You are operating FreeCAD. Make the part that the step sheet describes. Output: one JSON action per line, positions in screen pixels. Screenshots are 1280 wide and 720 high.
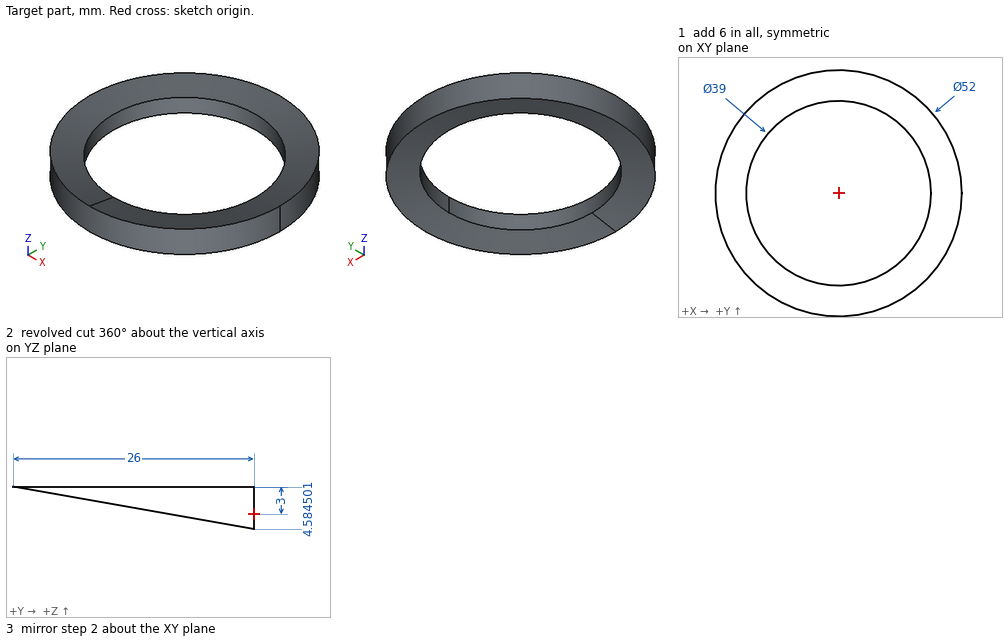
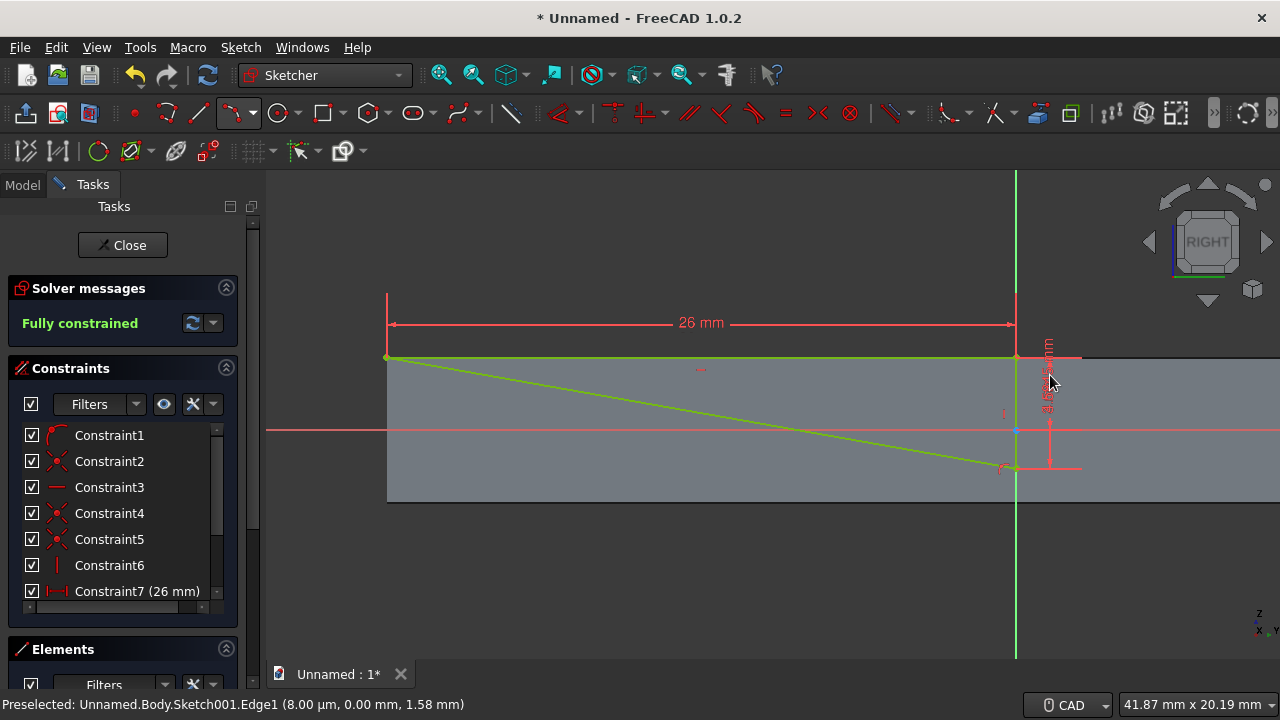
{"action": "left_click", "coordinate": [123, 245]}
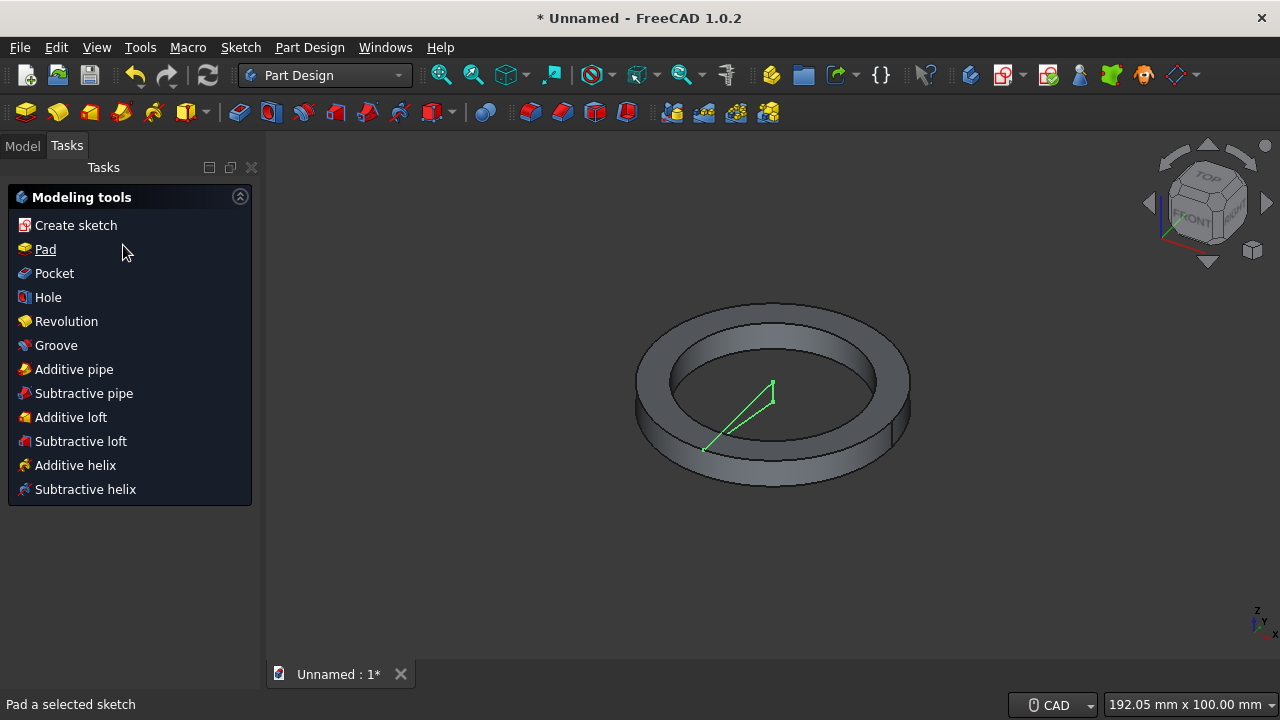
{"action": "left_click", "coordinate": [304, 112]}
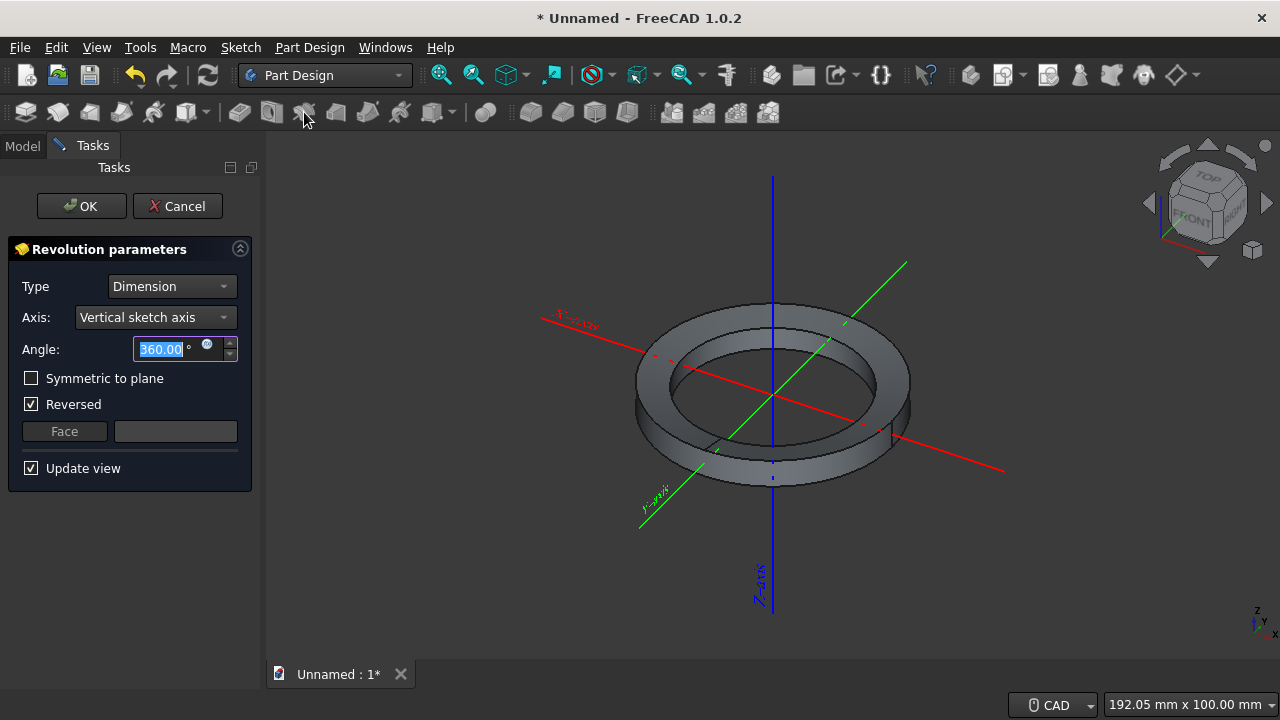
{"action": "left_click", "coordinate": [82, 206]}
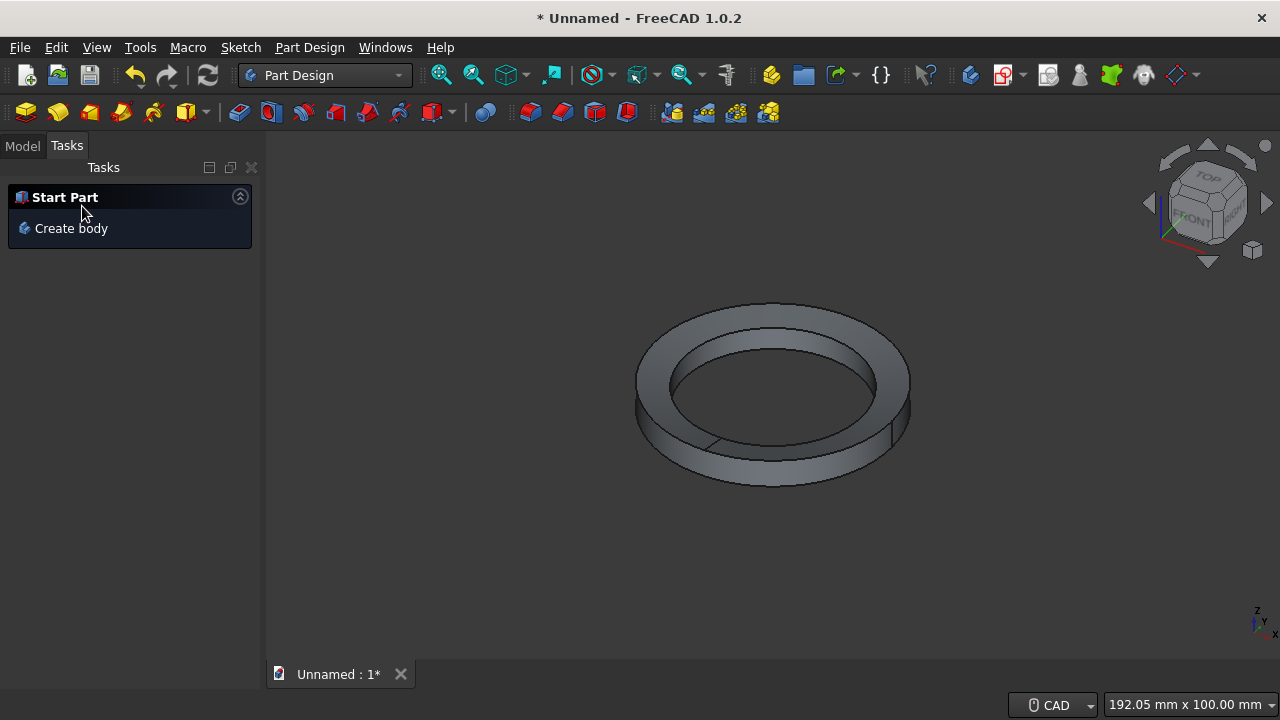
{"action": "left_click", "coordinate": [23, 145]}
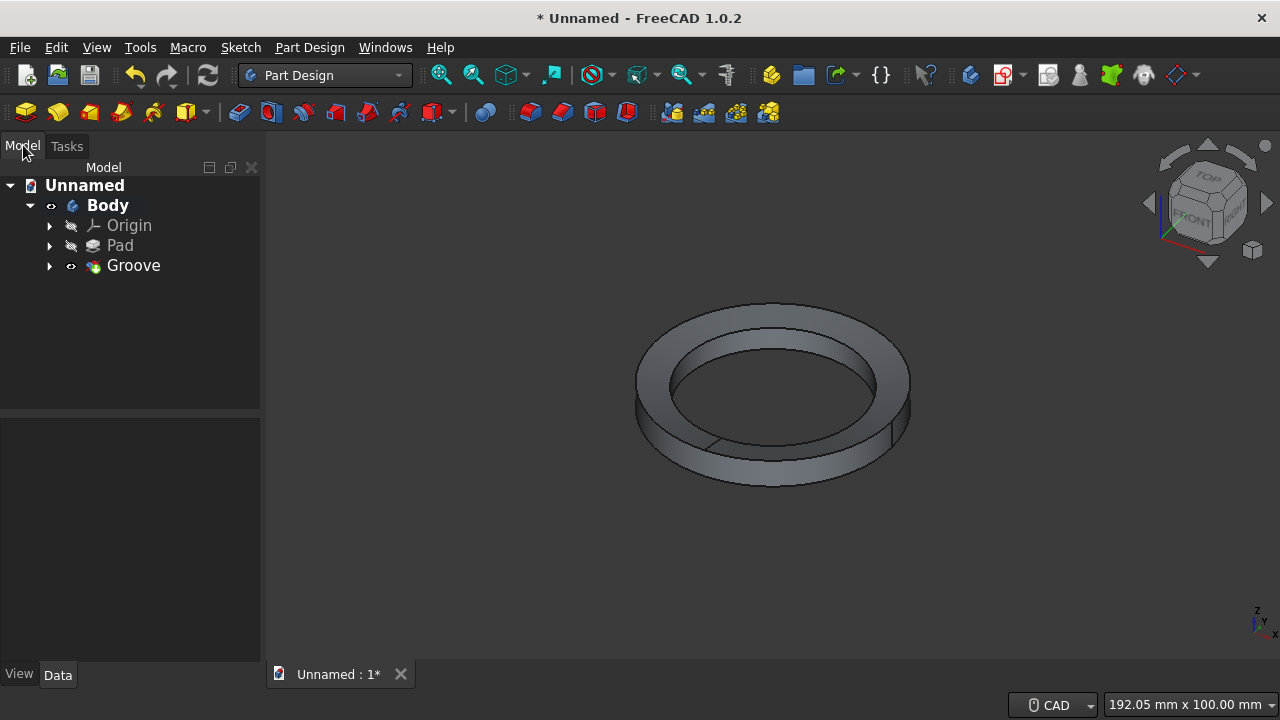
{"action": "left_click", "coordinate": [116, 266]}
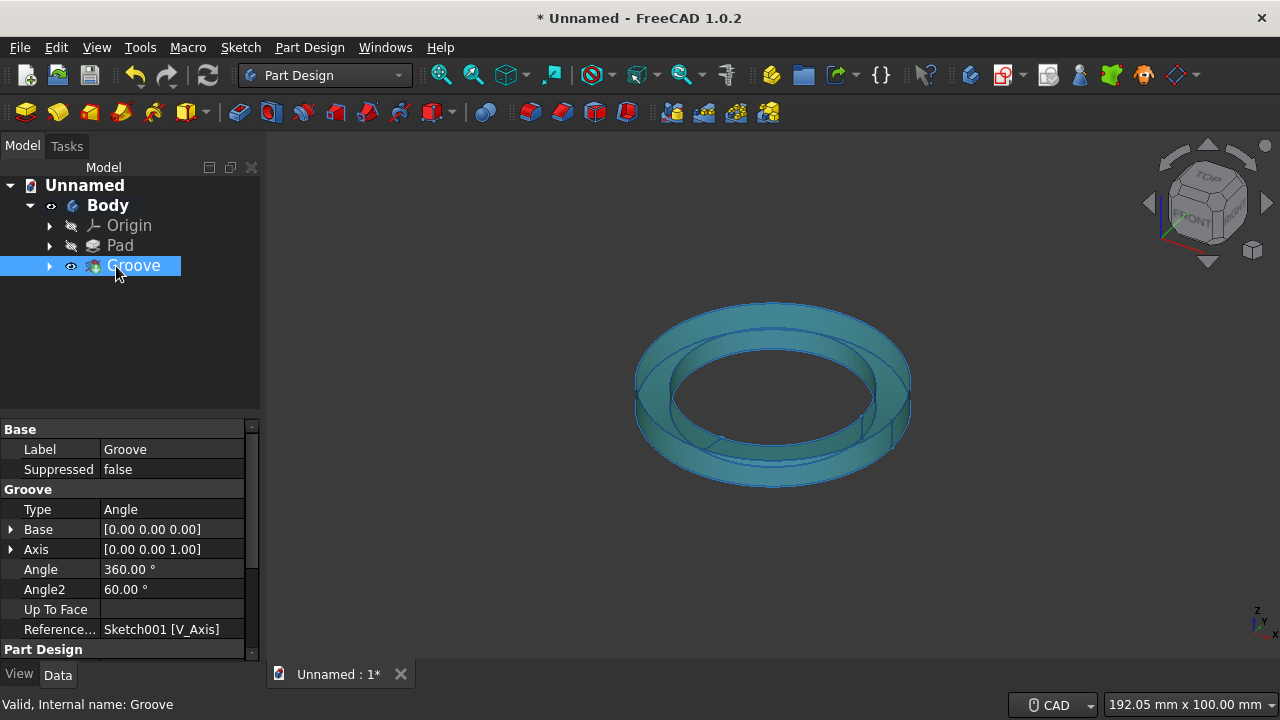
{"action": "left_click", "coordinate": [672, 112]}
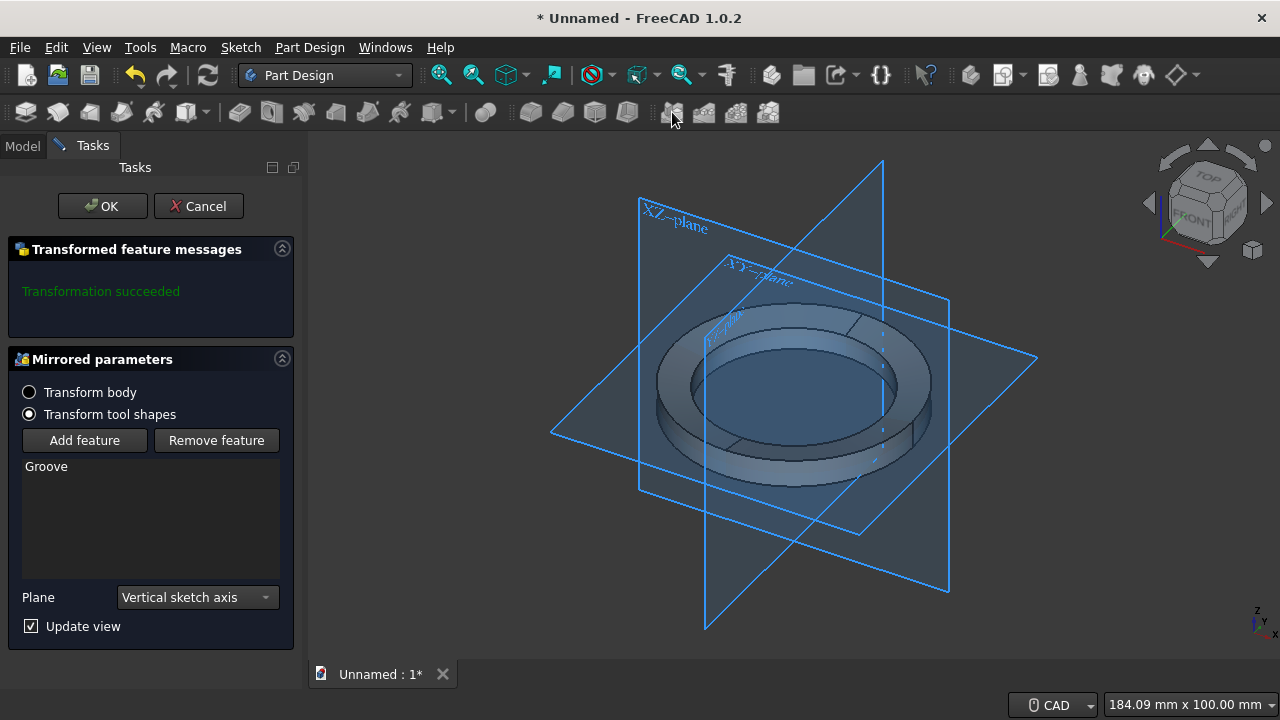
{"action": "left_click", "coordinate": [198, 598]}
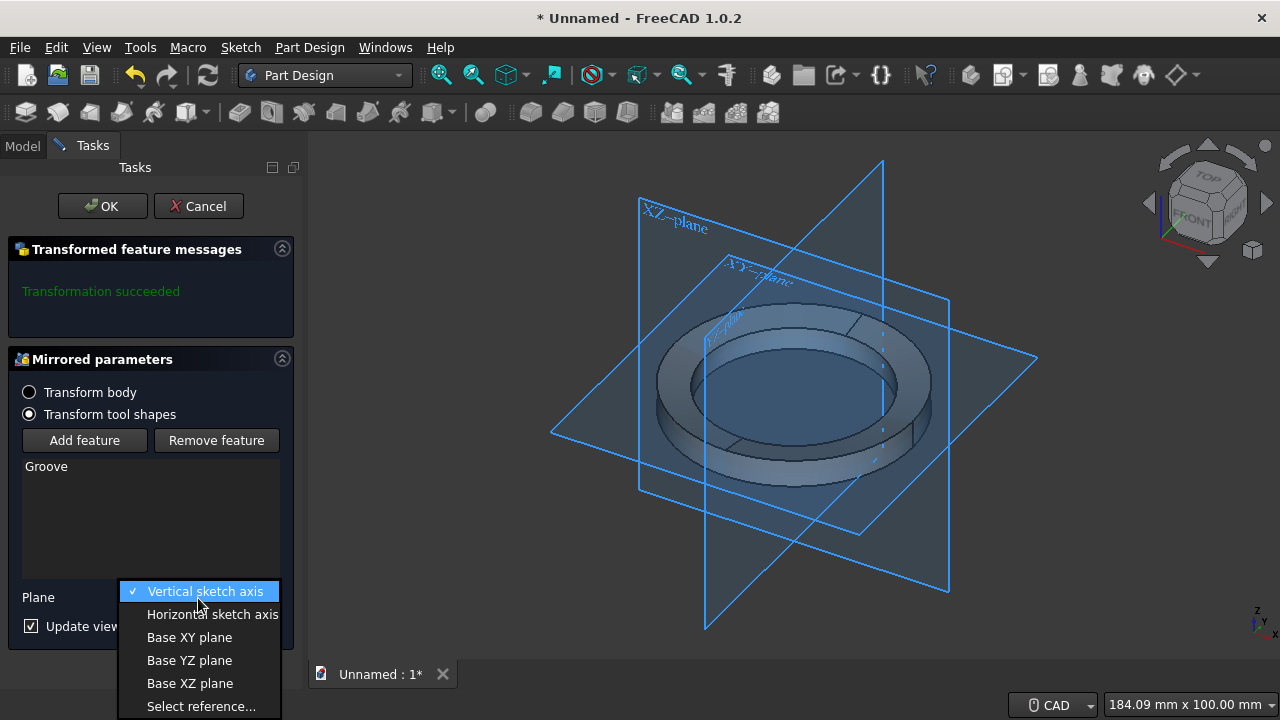
{"action": "left_click", "coordinate": [198, 638]}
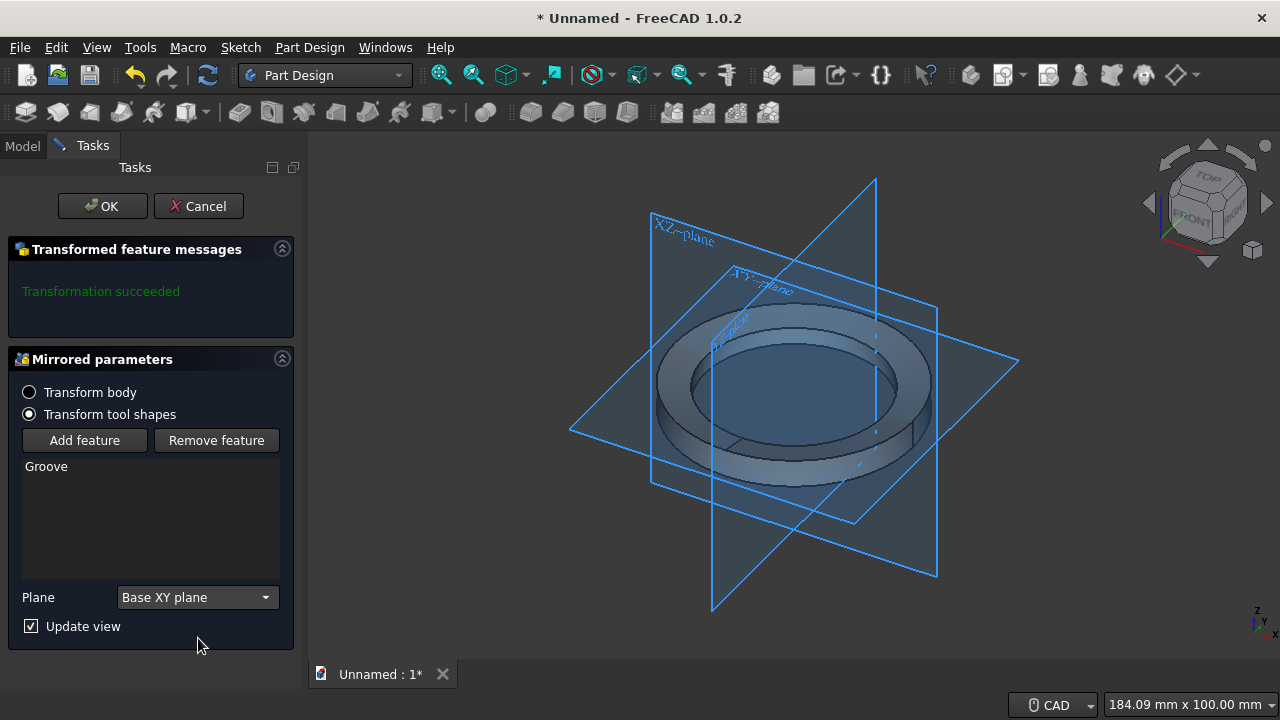
{"action": "left_click", "coordinate": [103, 206]}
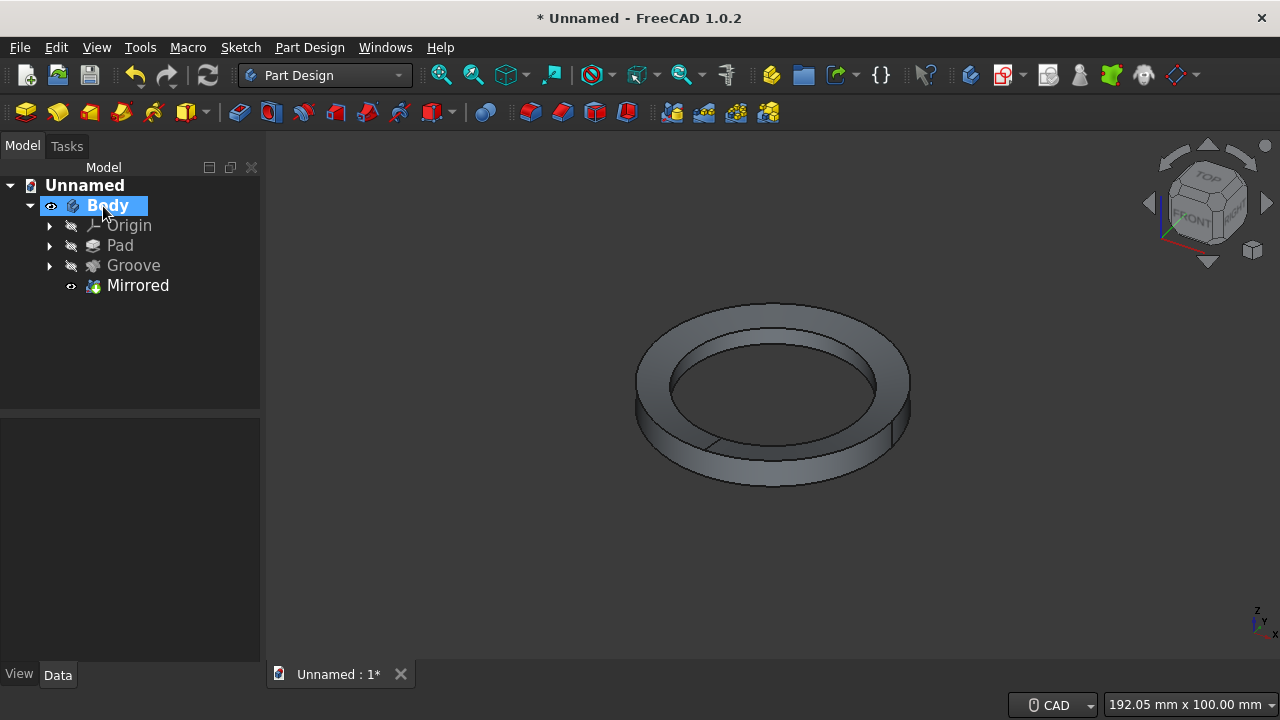
{"action": "key", "text": "0"}